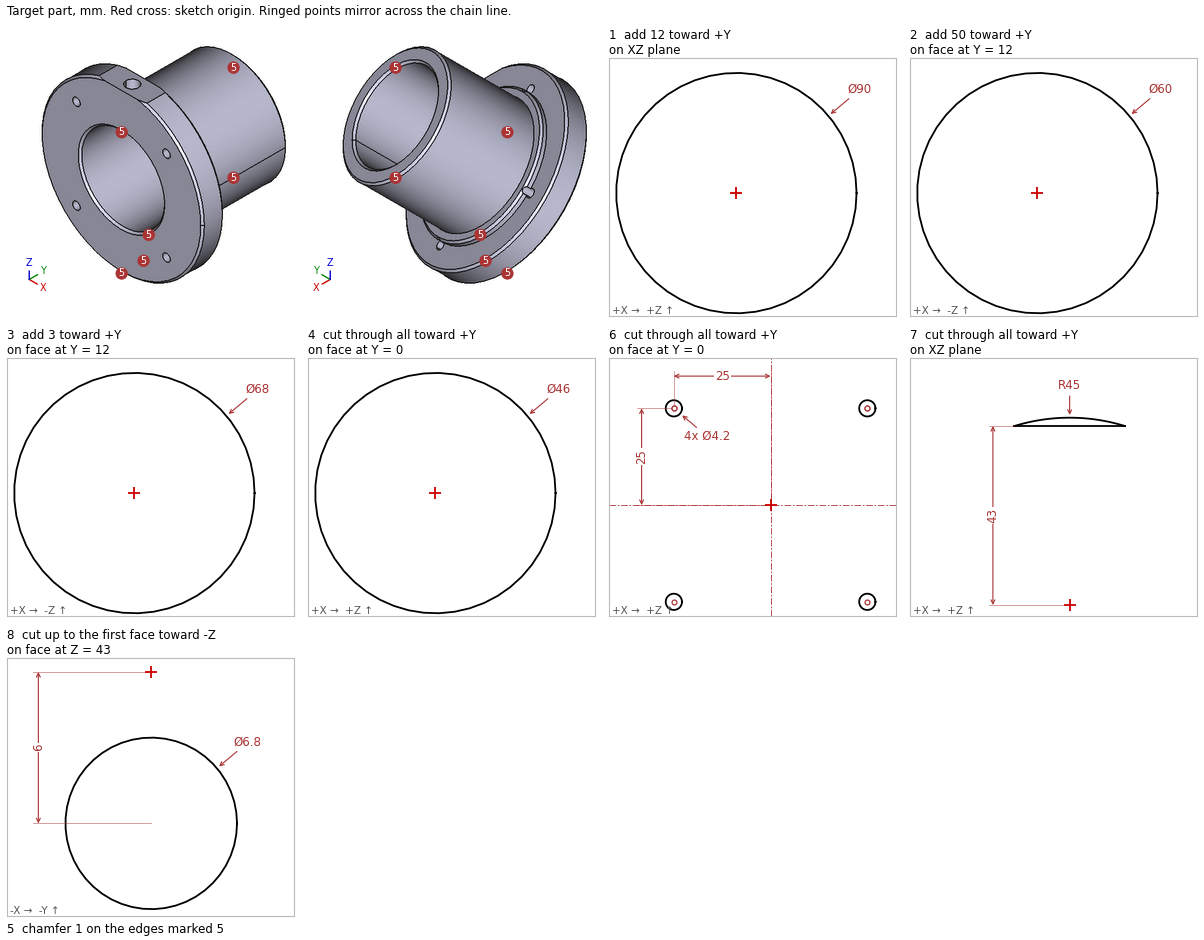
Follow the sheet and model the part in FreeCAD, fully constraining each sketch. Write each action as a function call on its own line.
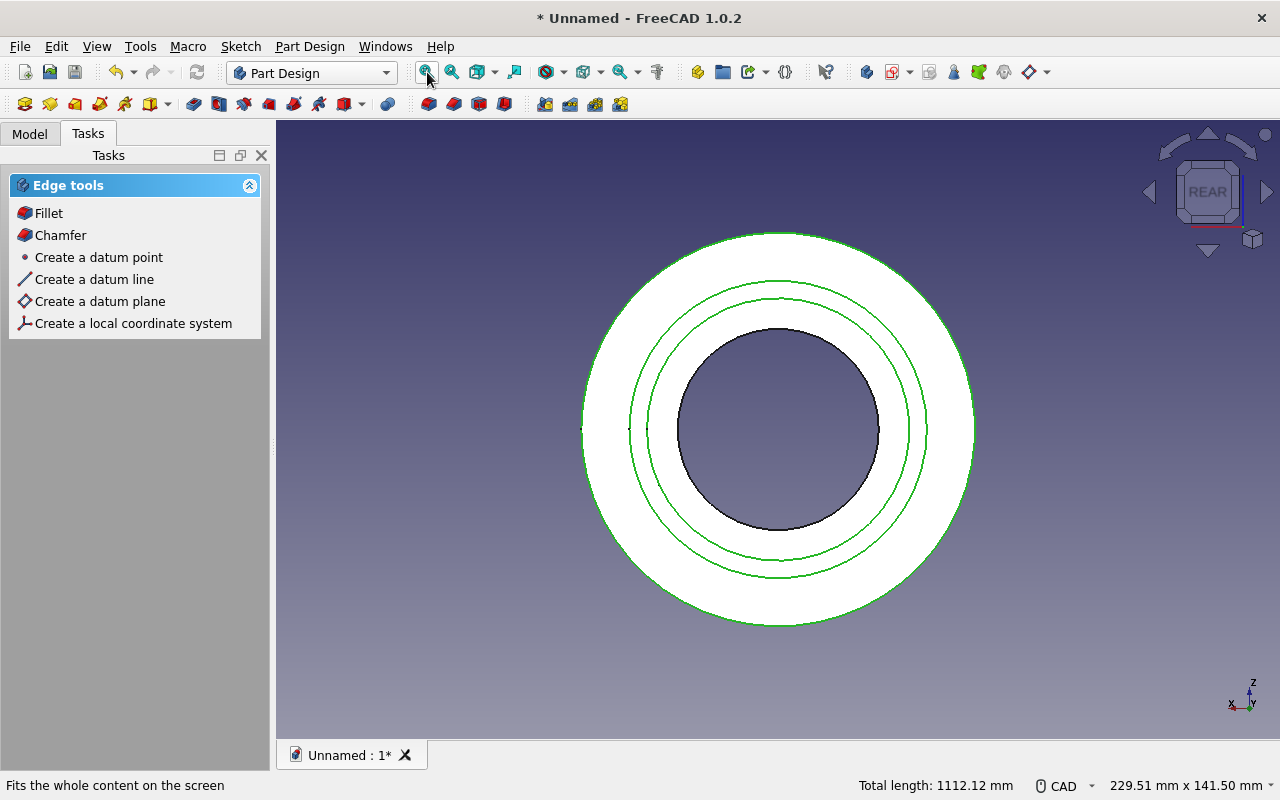
click(860, 369, ctrl)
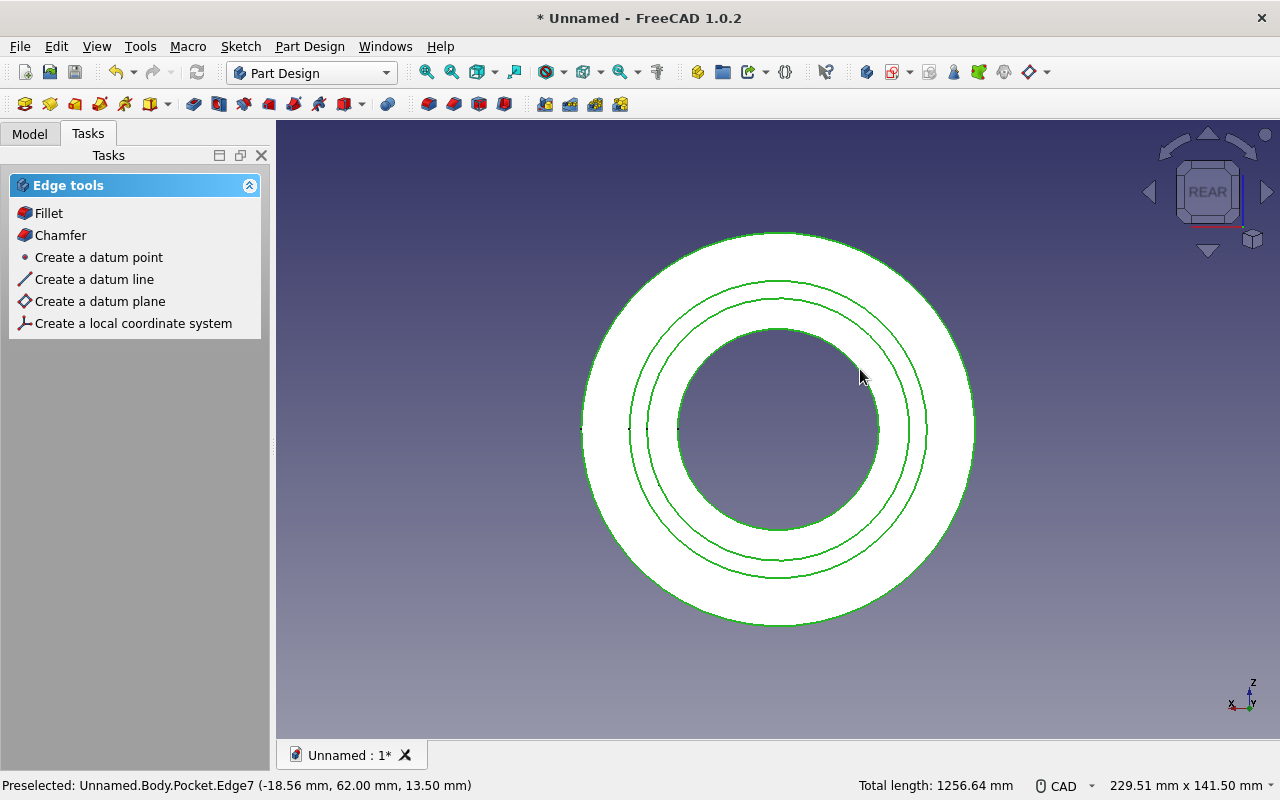
click(454, 104)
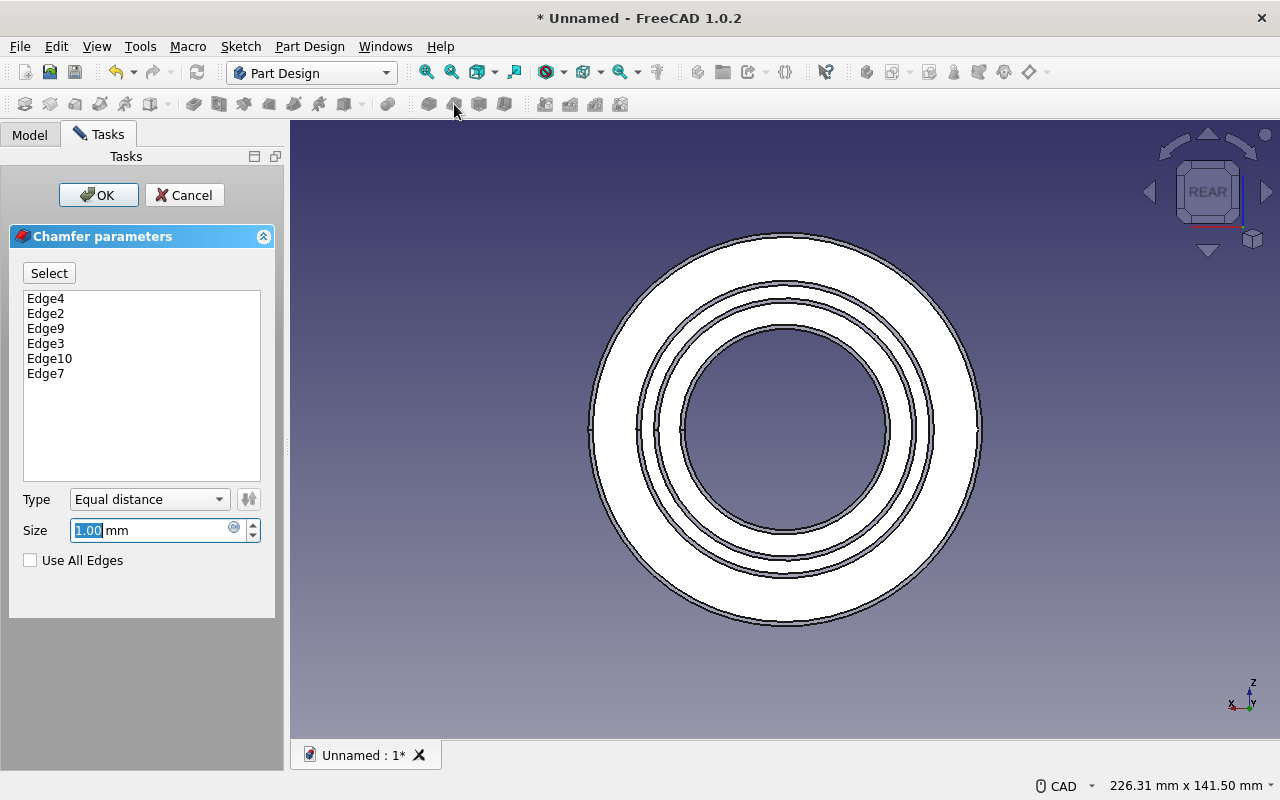
text(1)
key(Tab)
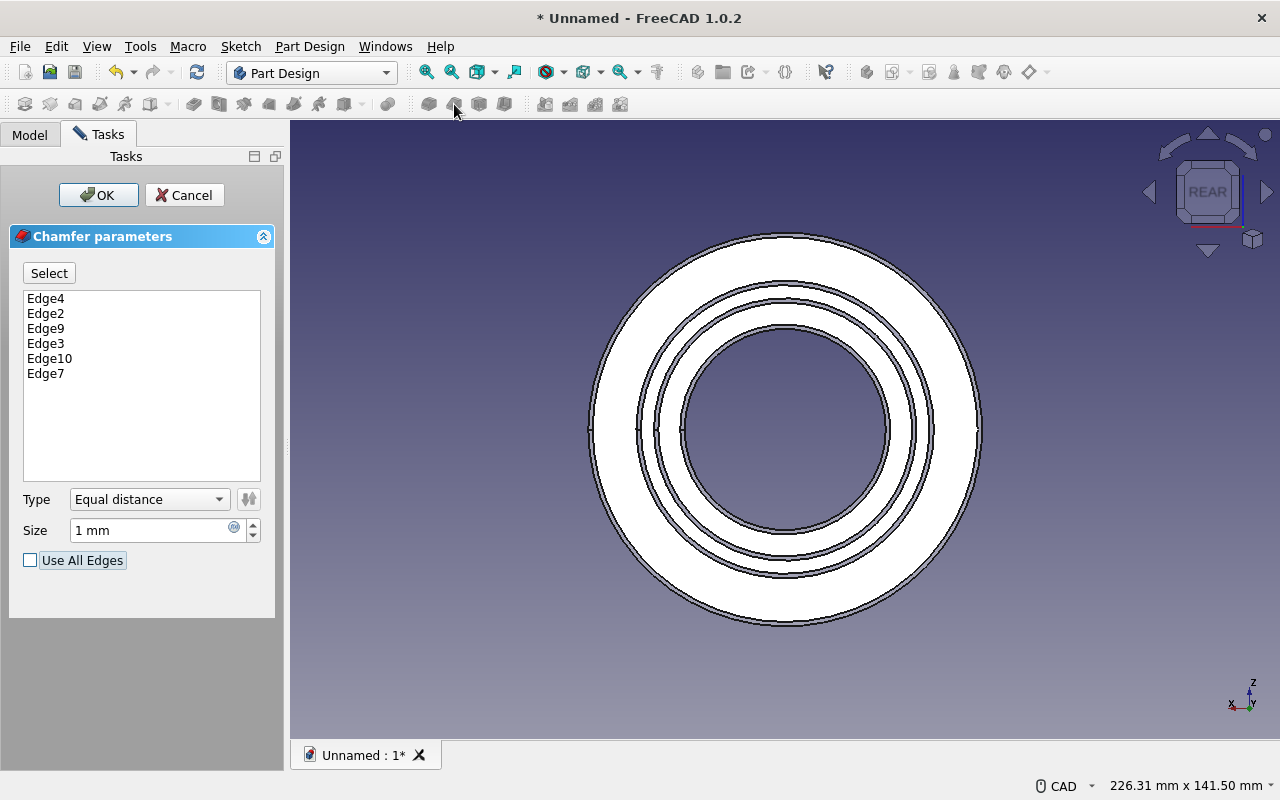
click(99, 195)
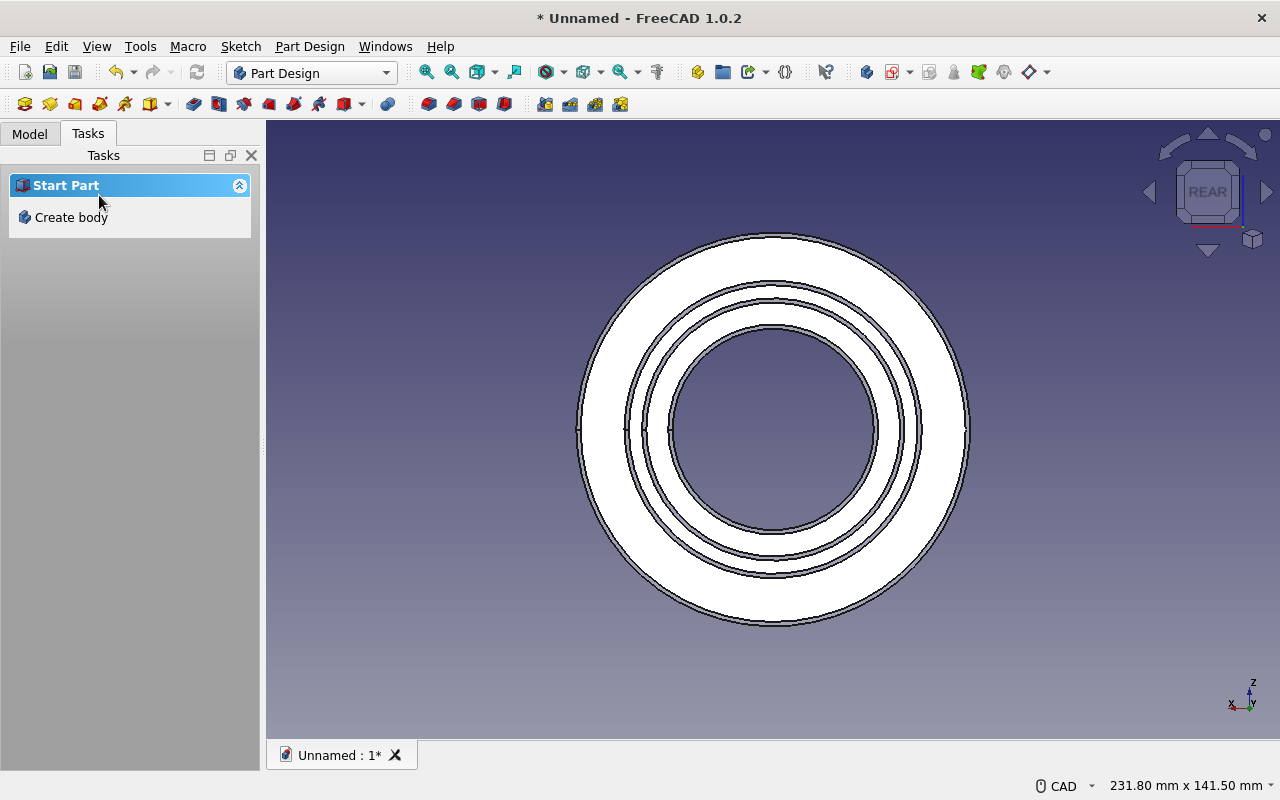
key(0)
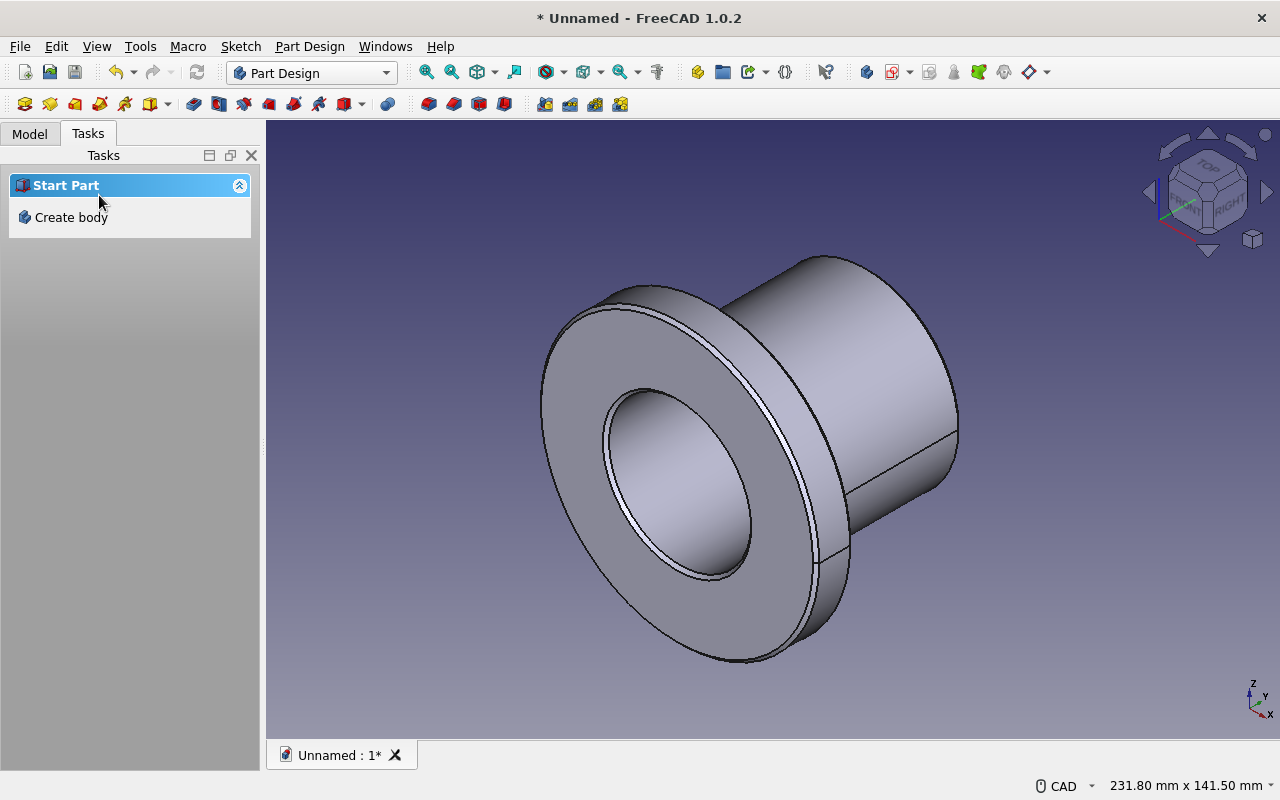
click(599, 529)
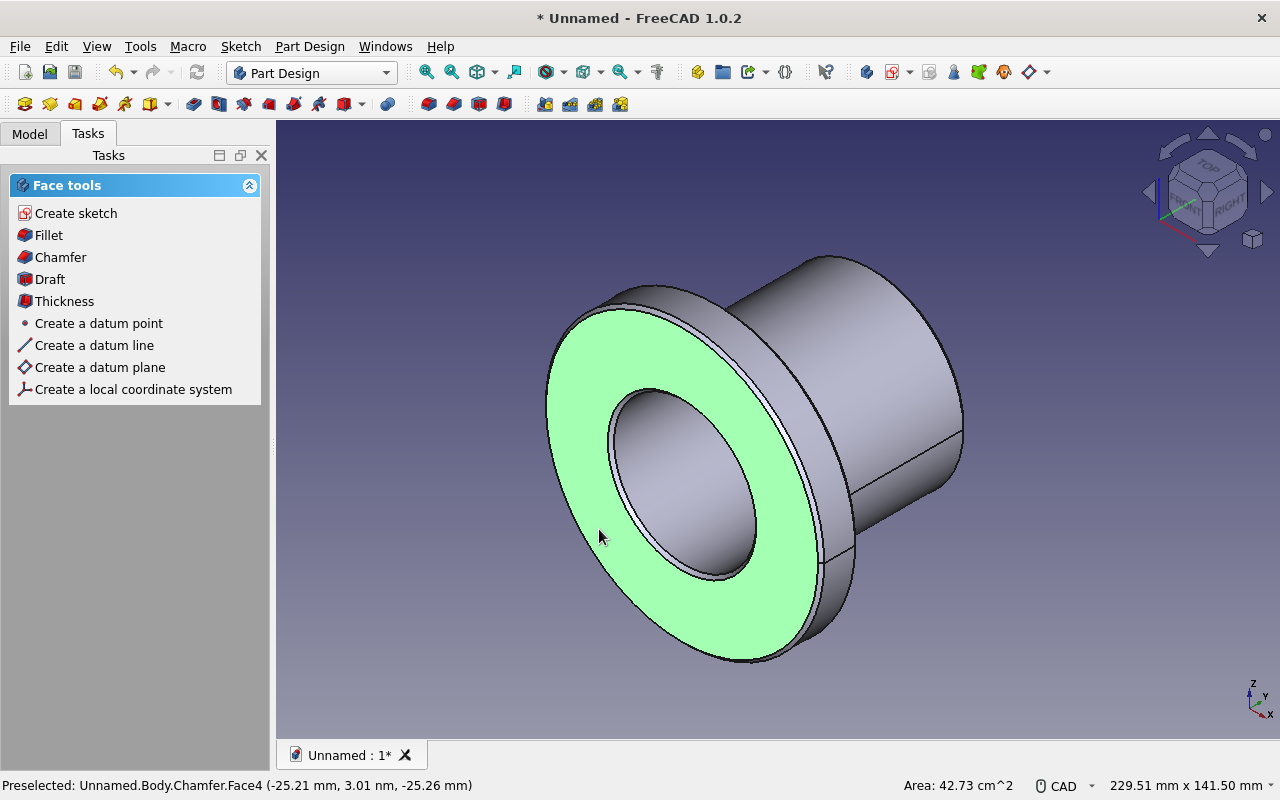
click(892, 72)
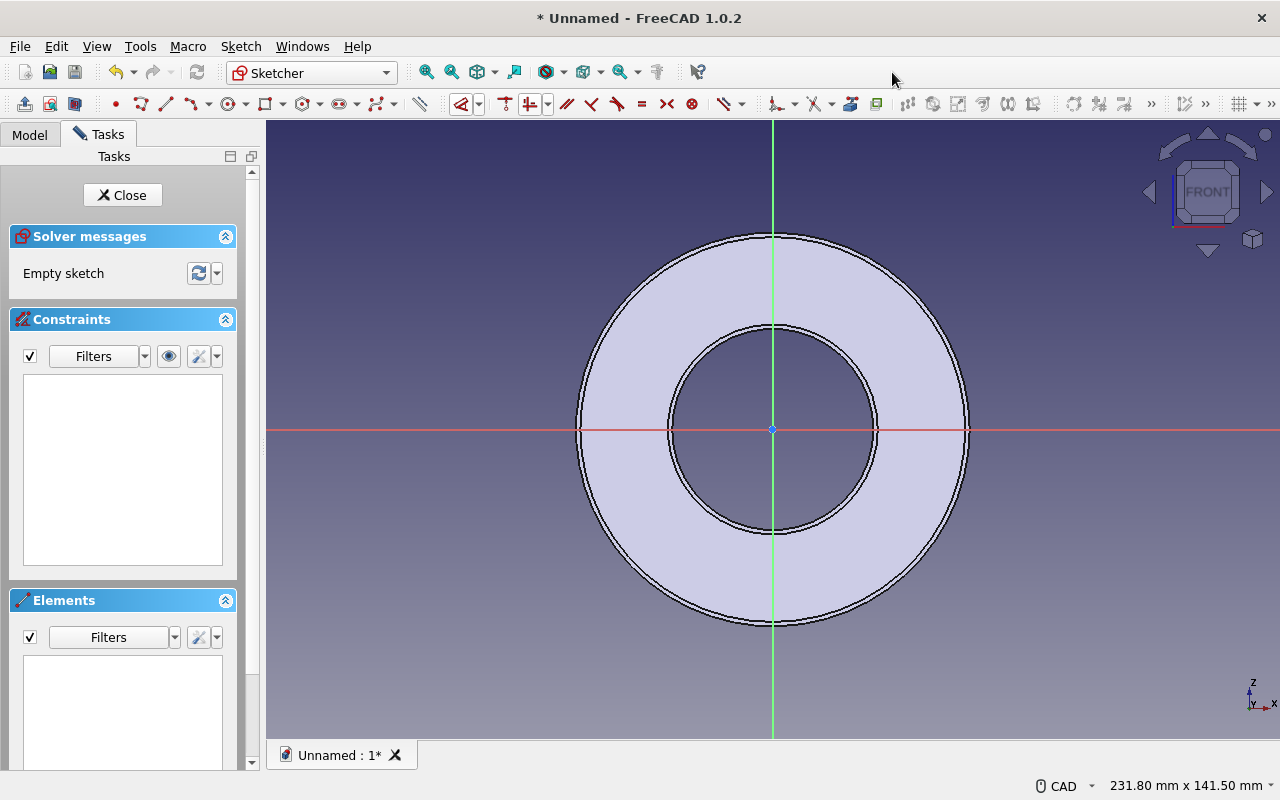
scroll(856, 429, up, 3)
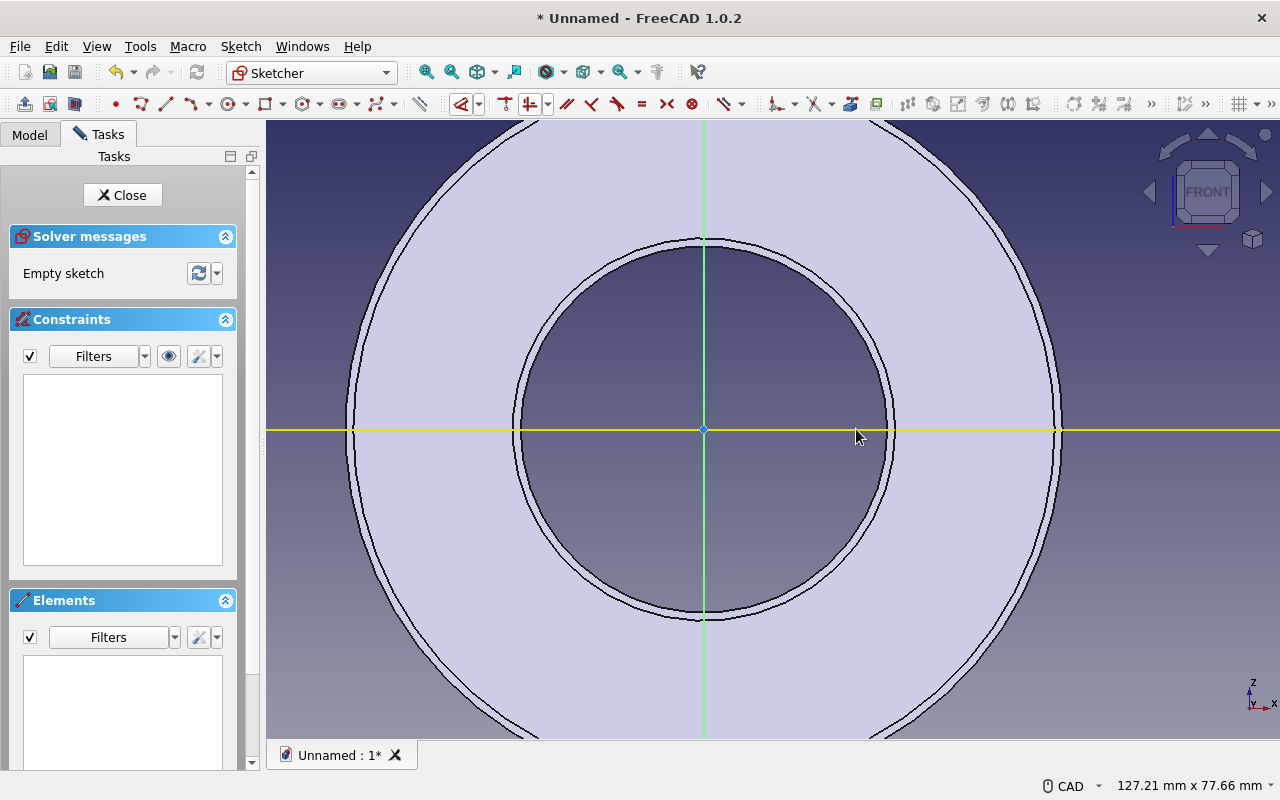
click(228, 104)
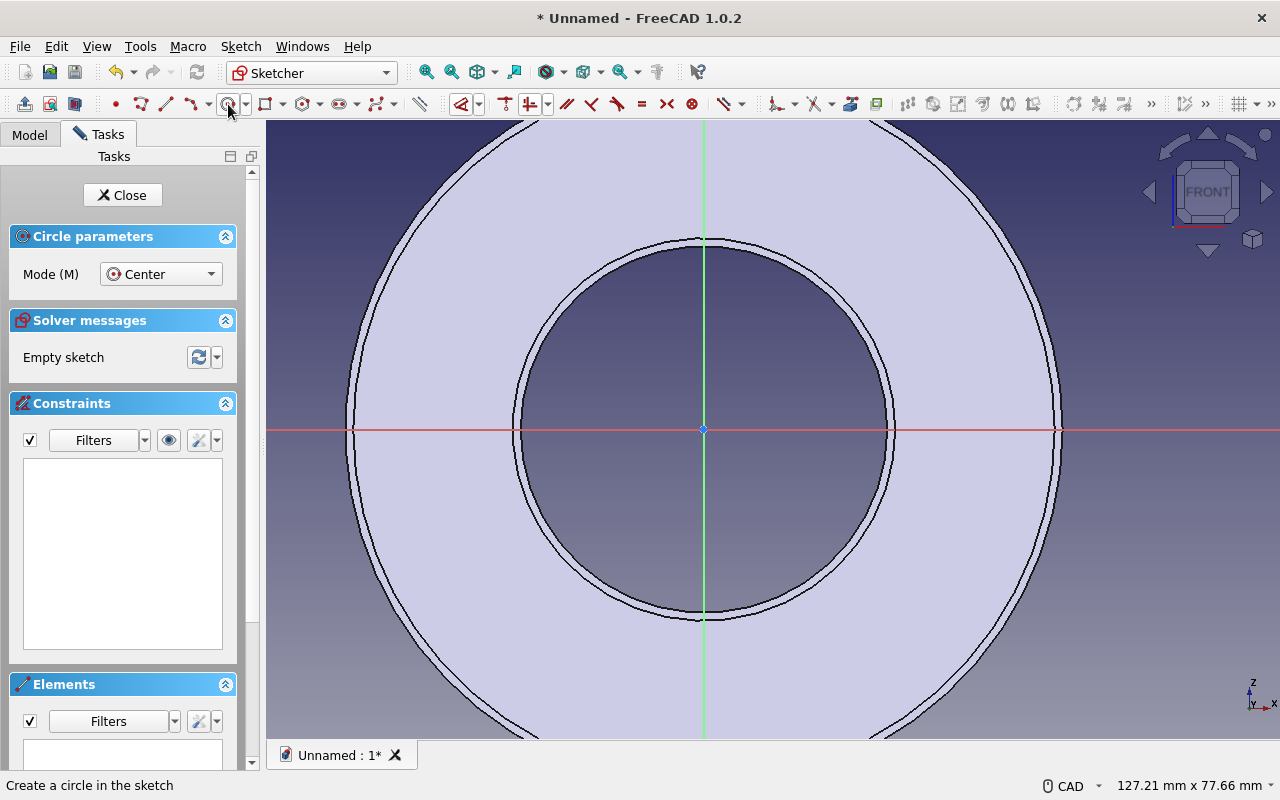
scroll(505, 230, up, 2)